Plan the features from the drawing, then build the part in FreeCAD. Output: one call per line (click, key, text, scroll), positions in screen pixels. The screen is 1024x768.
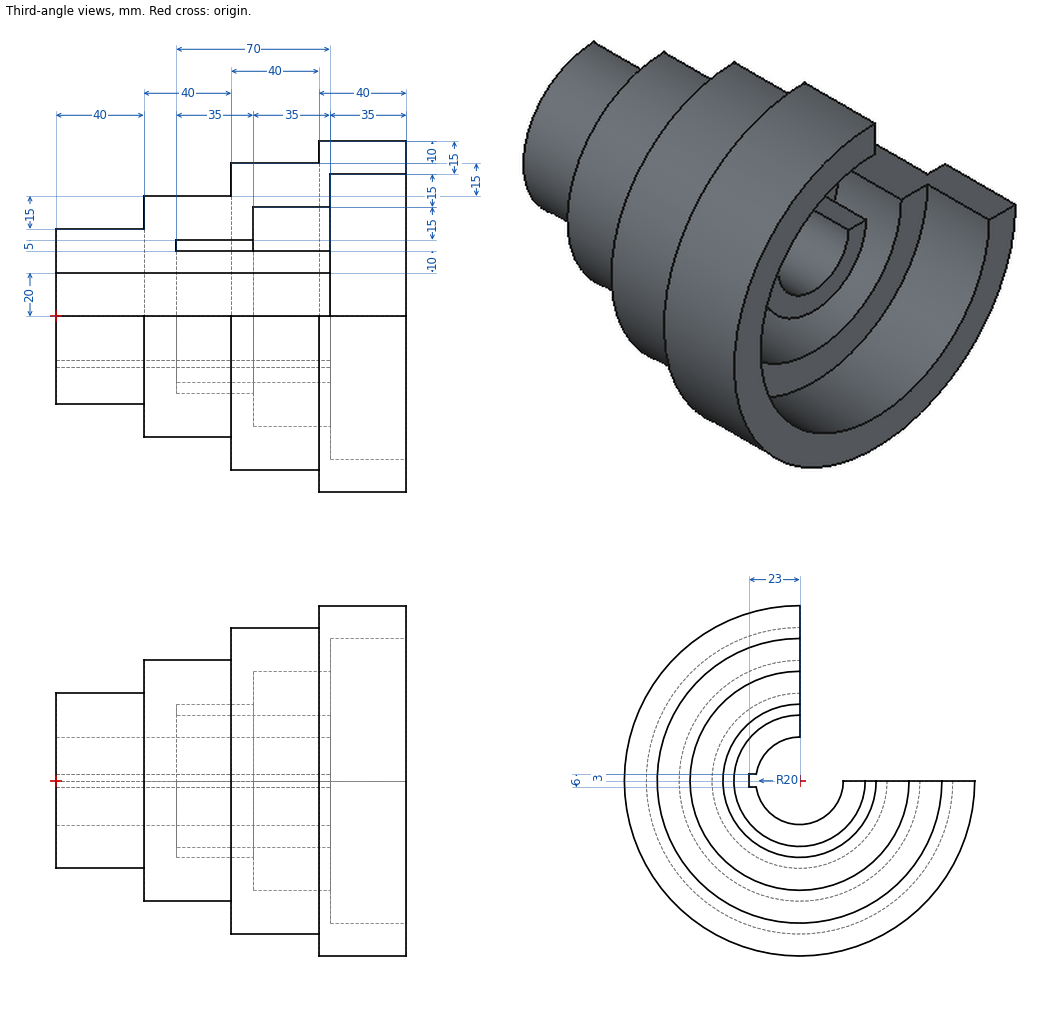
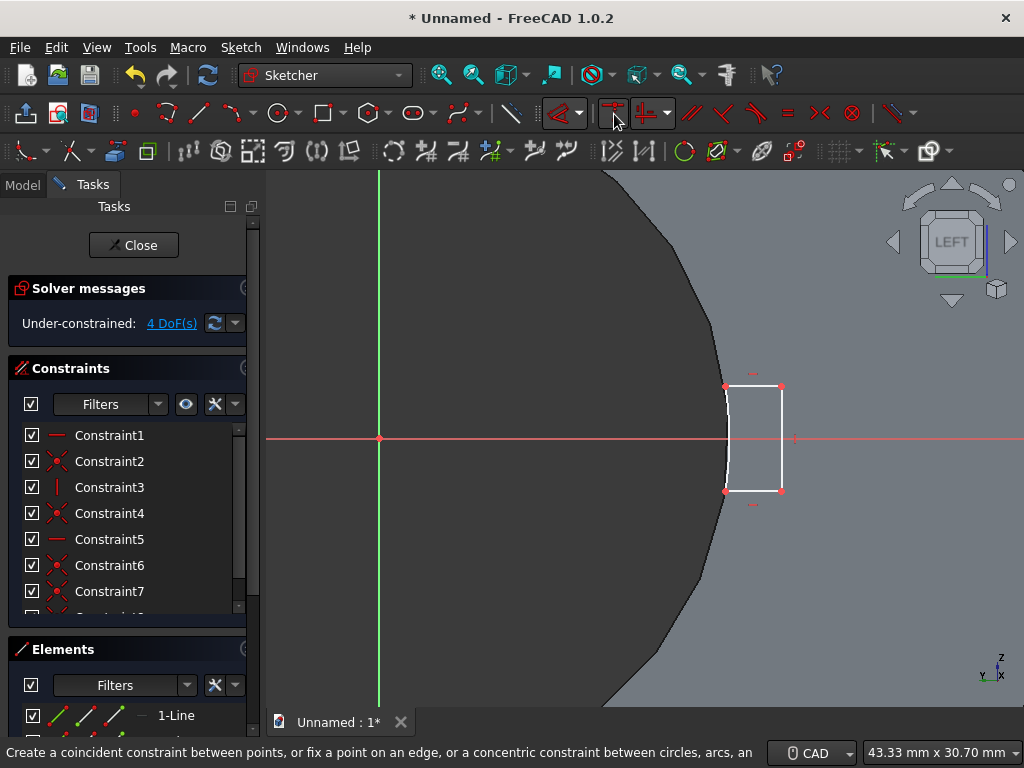
click(729, 460)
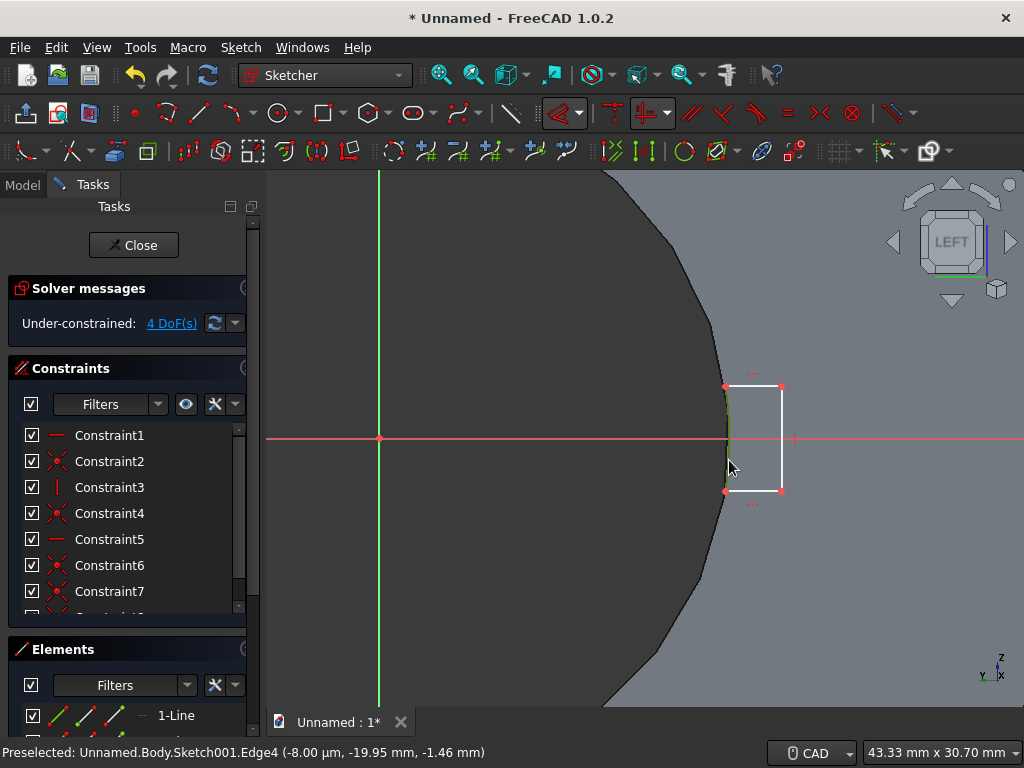
click(582, 114)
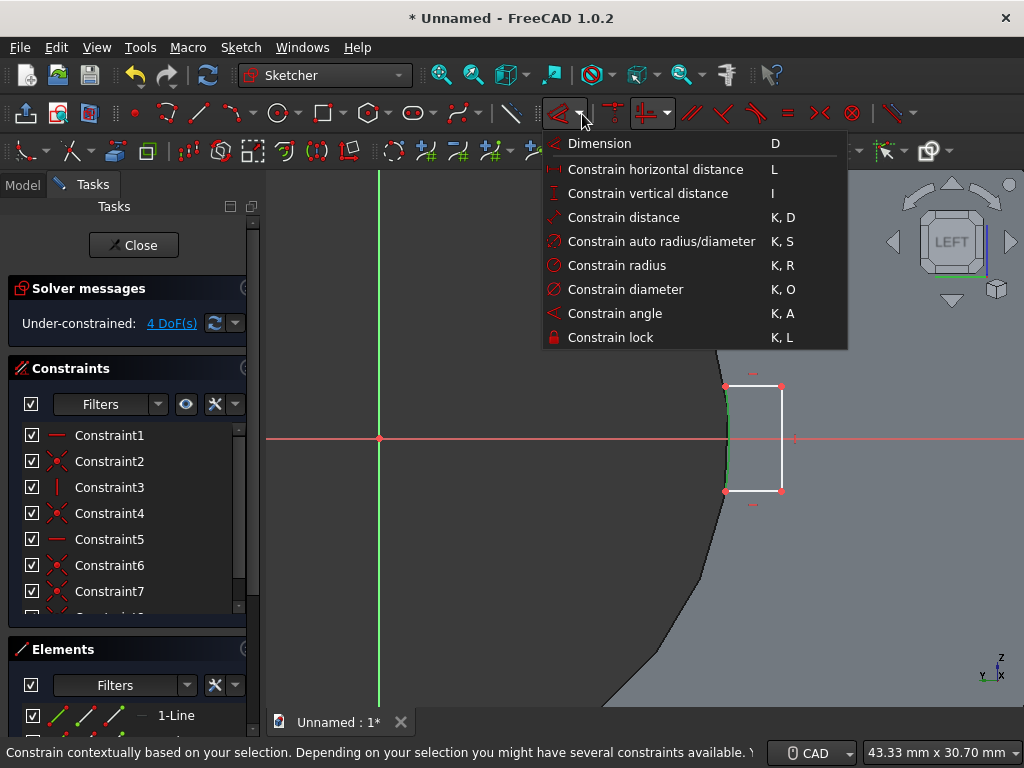
click(695, 265)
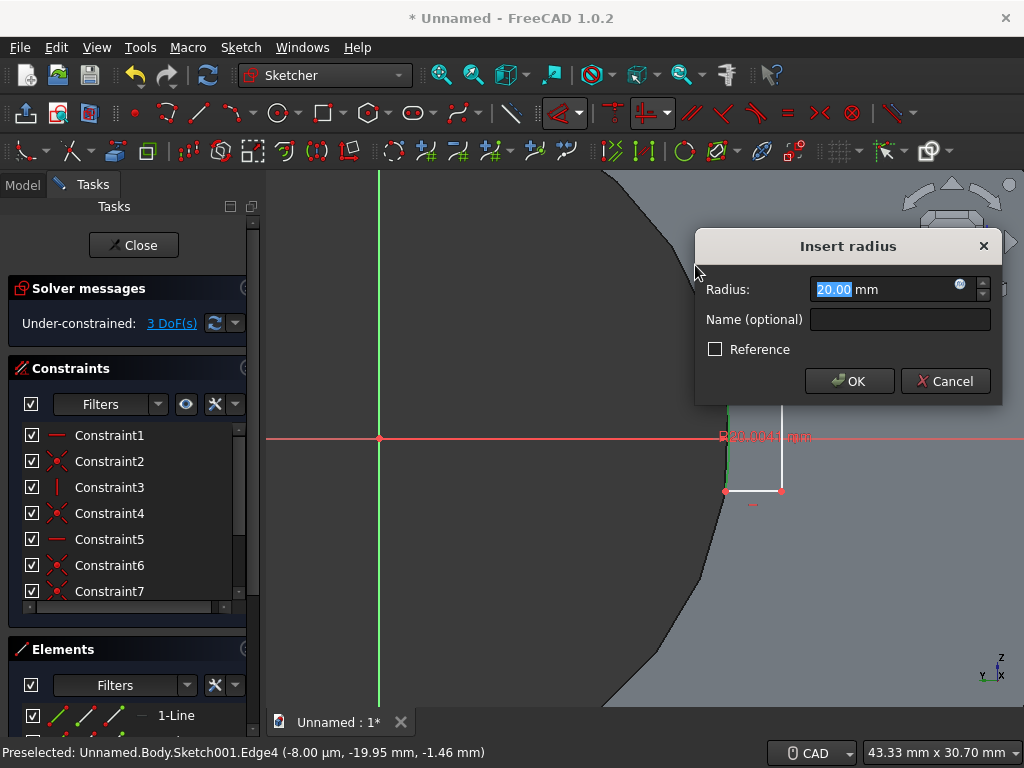
text(20)
key(Return)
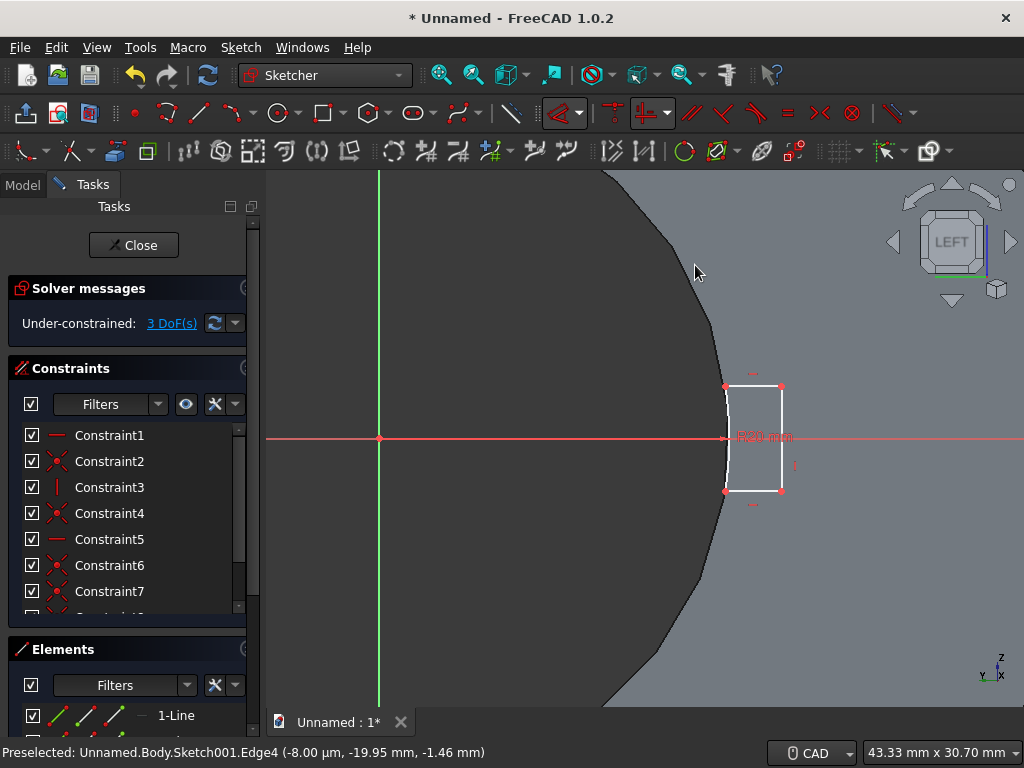
click(782, 418)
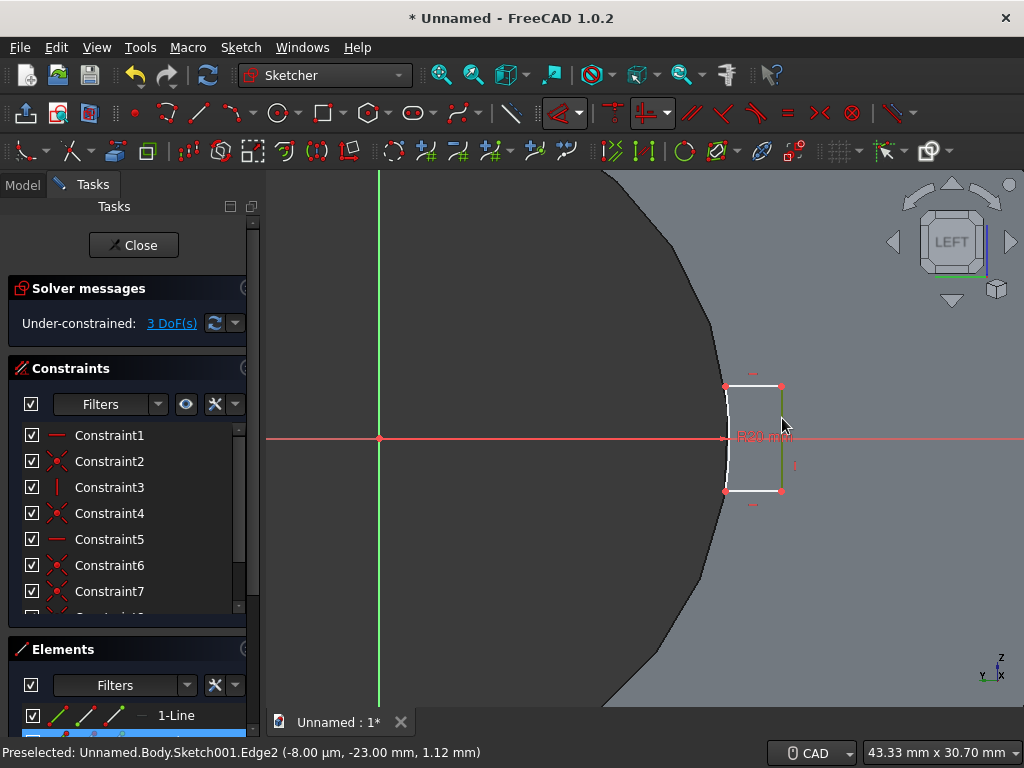
click(582, 114)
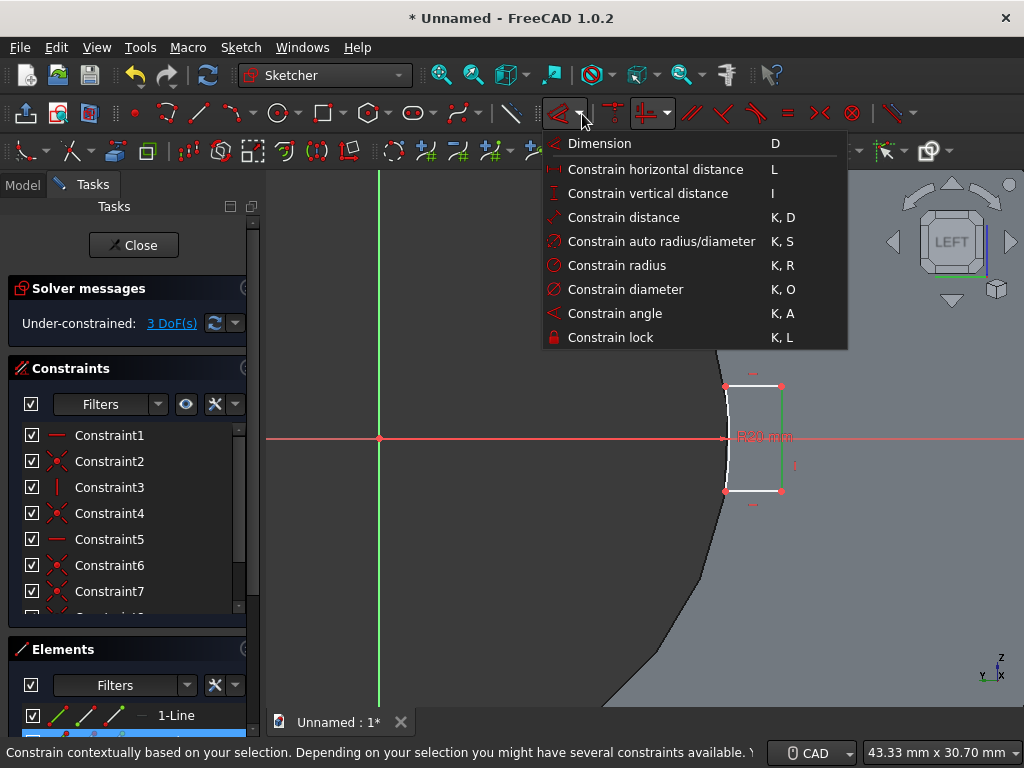
click(695, 193)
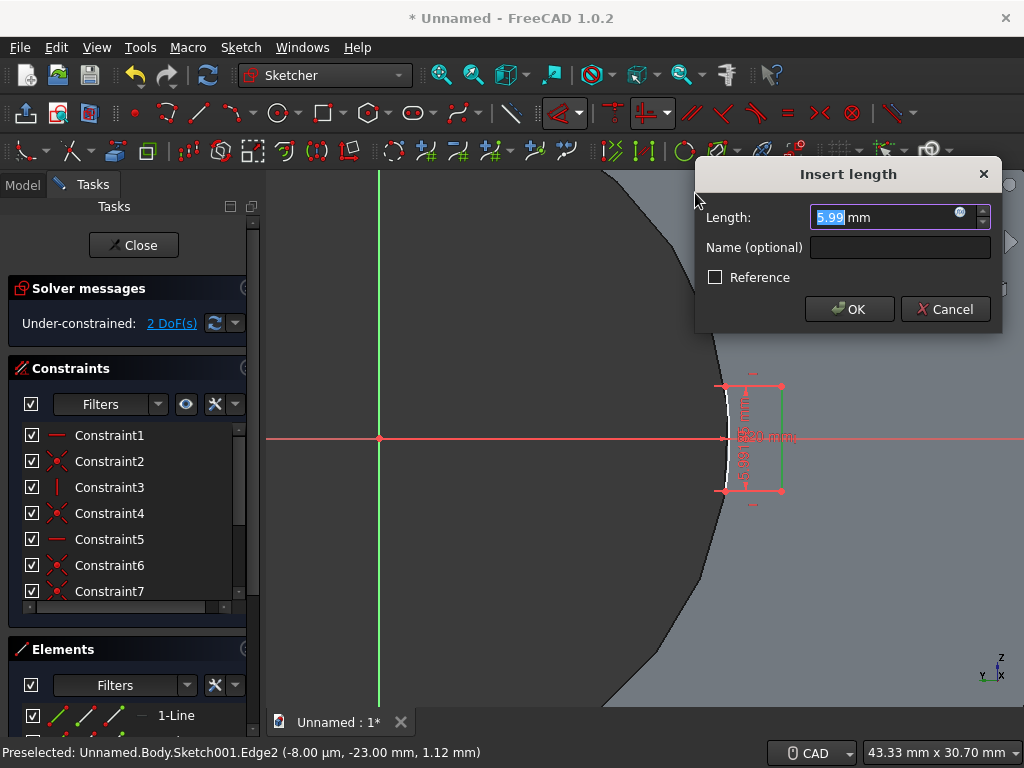
text(6)
key(Return)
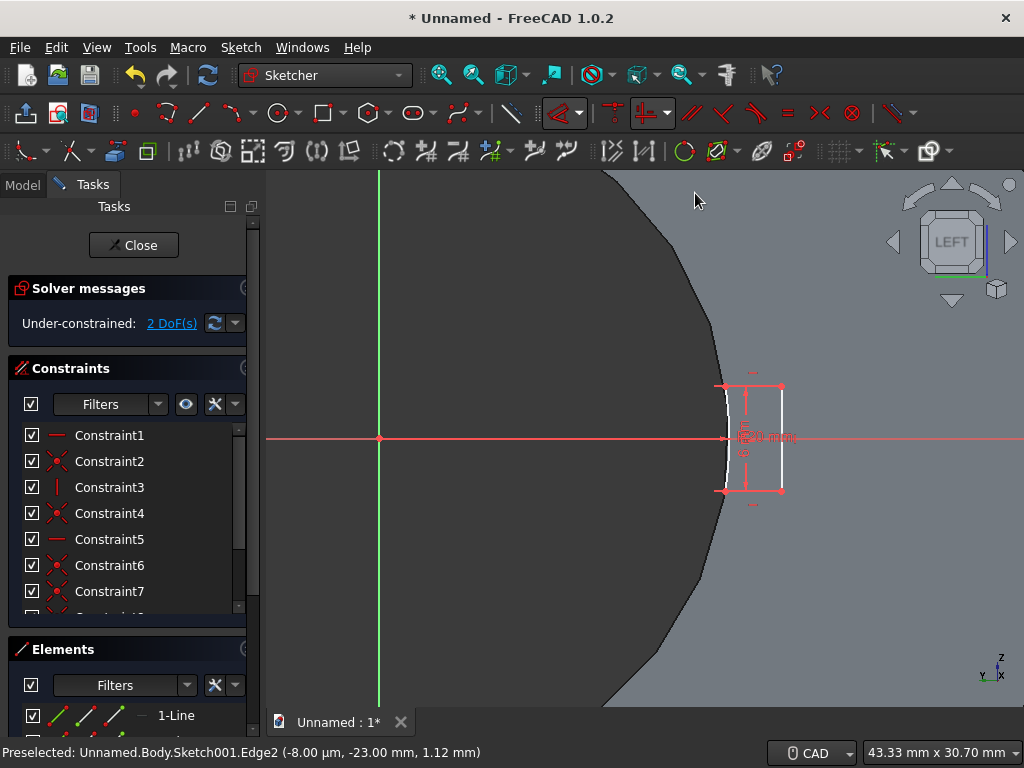
click(725, 386)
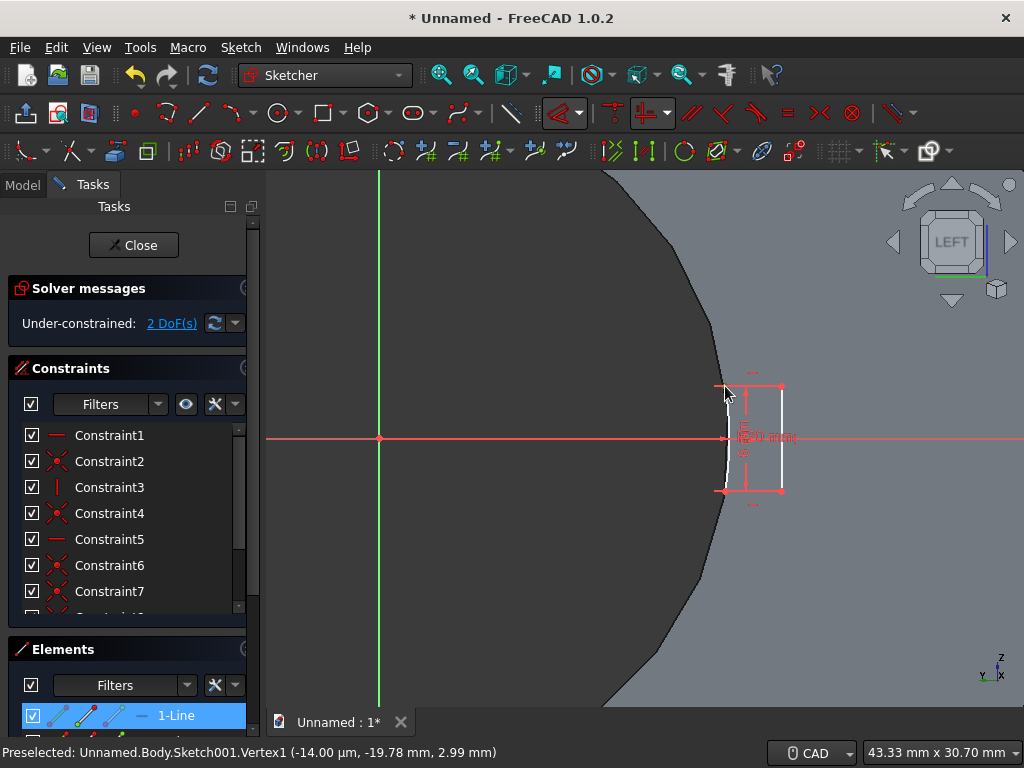
key(i)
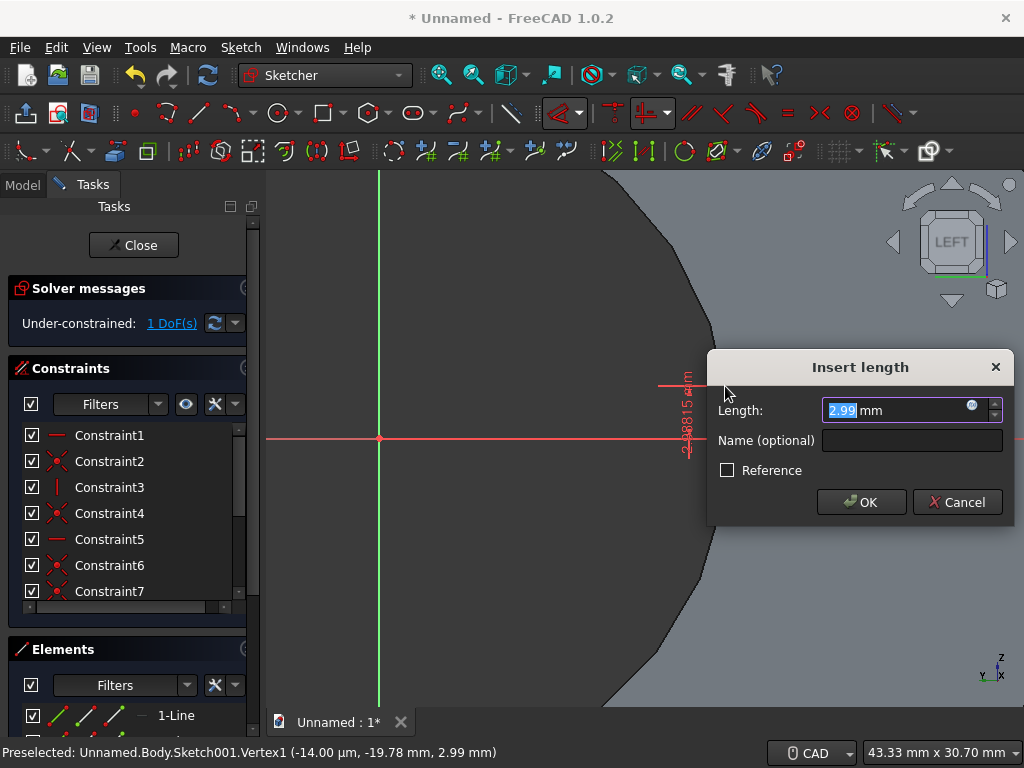
text(3)
key(Return)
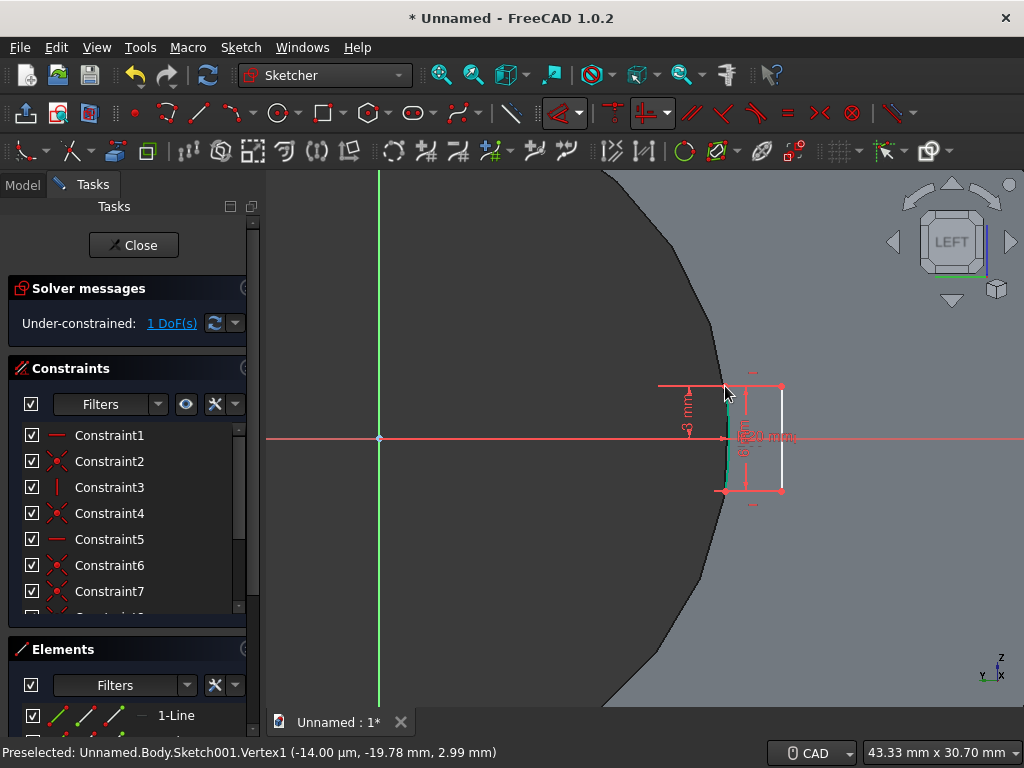
click(782, 386)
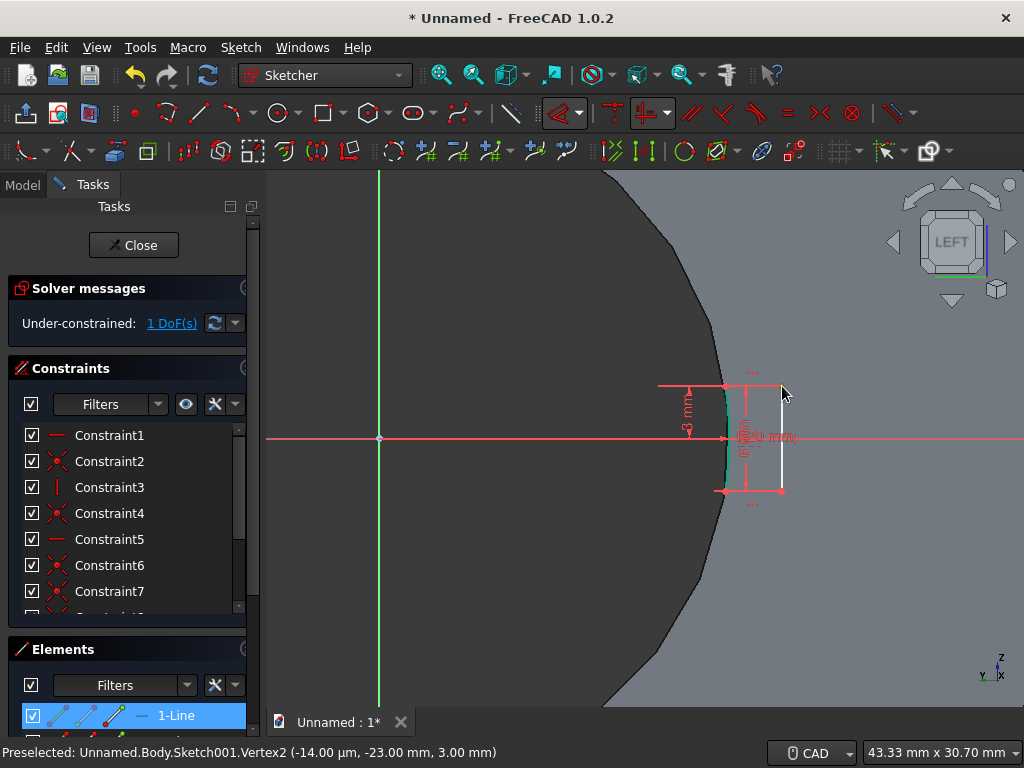
click(582, 114)